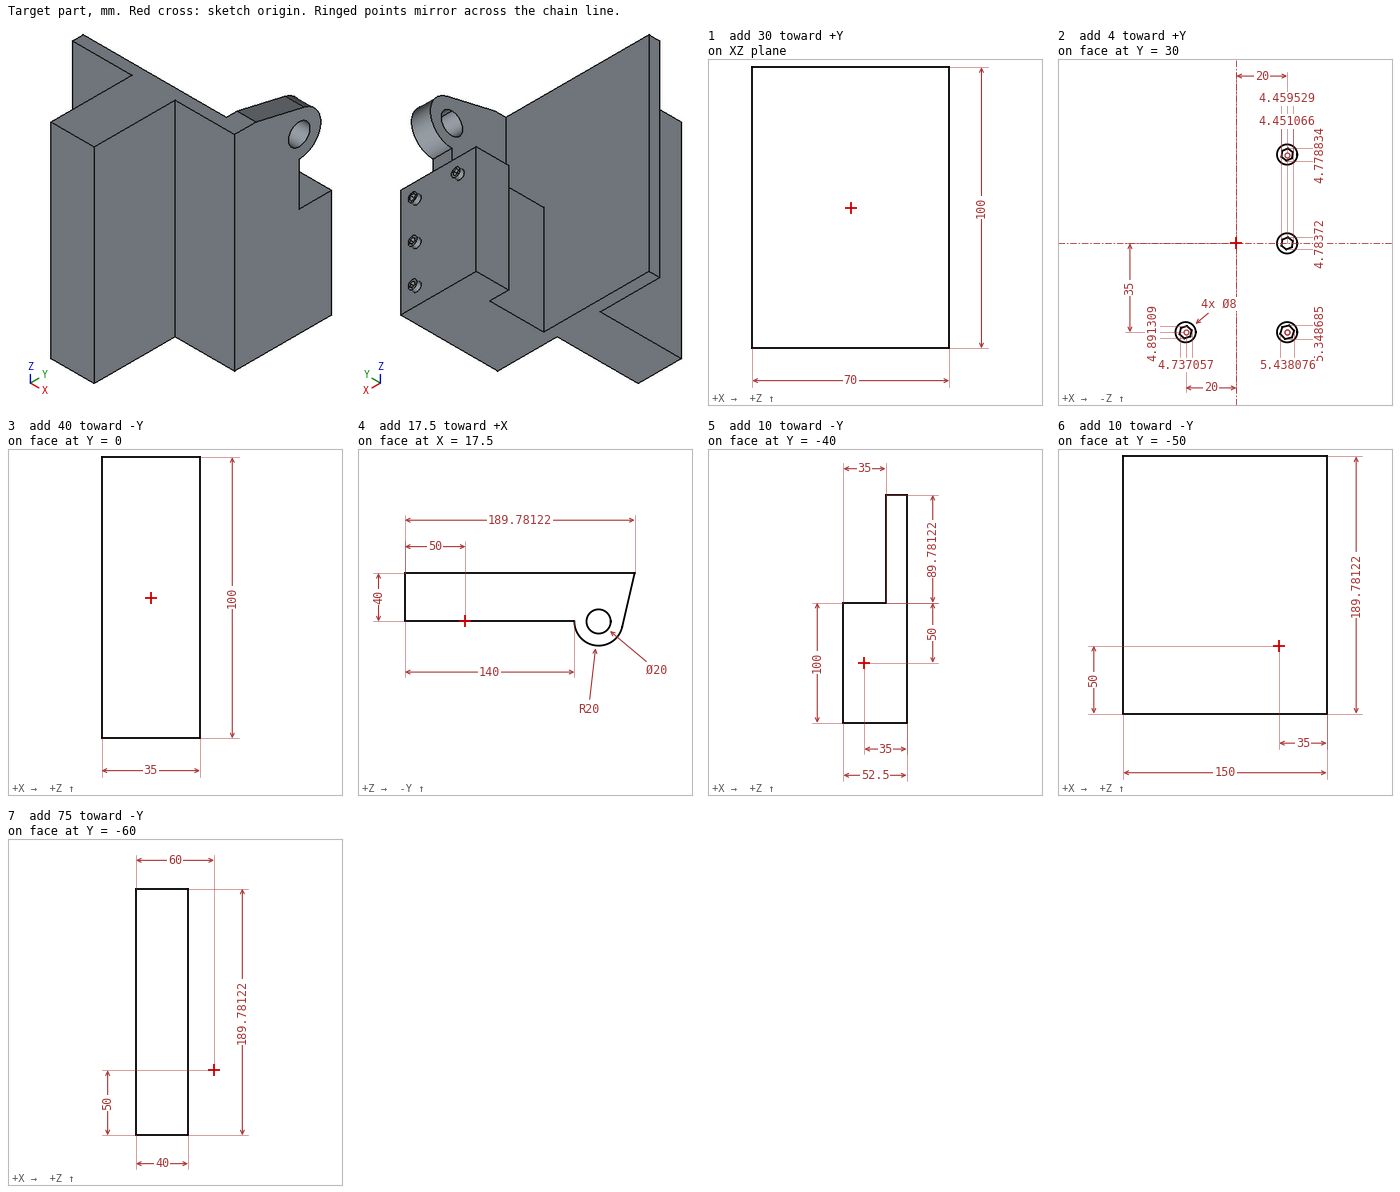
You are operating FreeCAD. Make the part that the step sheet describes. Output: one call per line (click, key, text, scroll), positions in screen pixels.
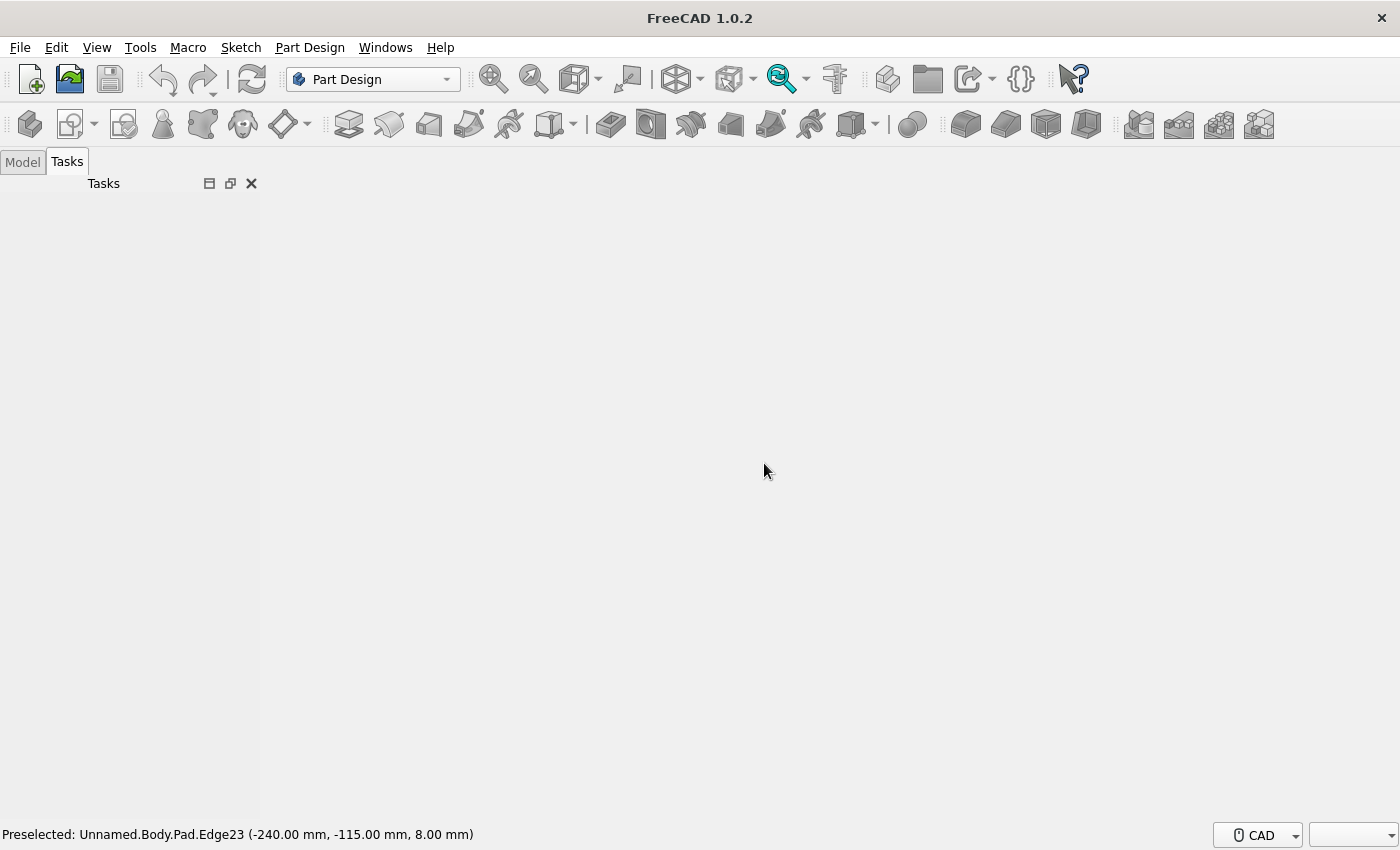
key(ctrl+n)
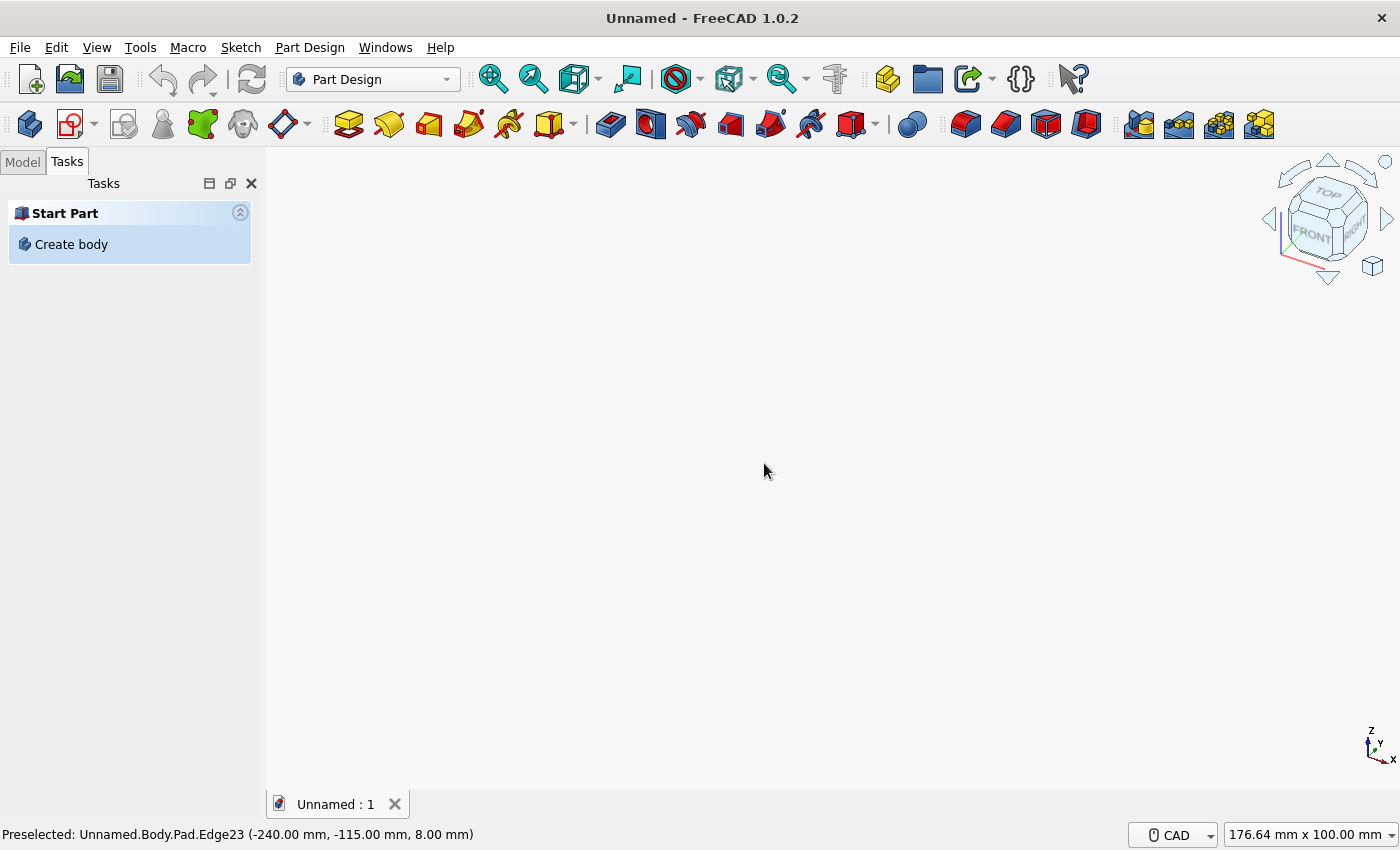
click(70, 124)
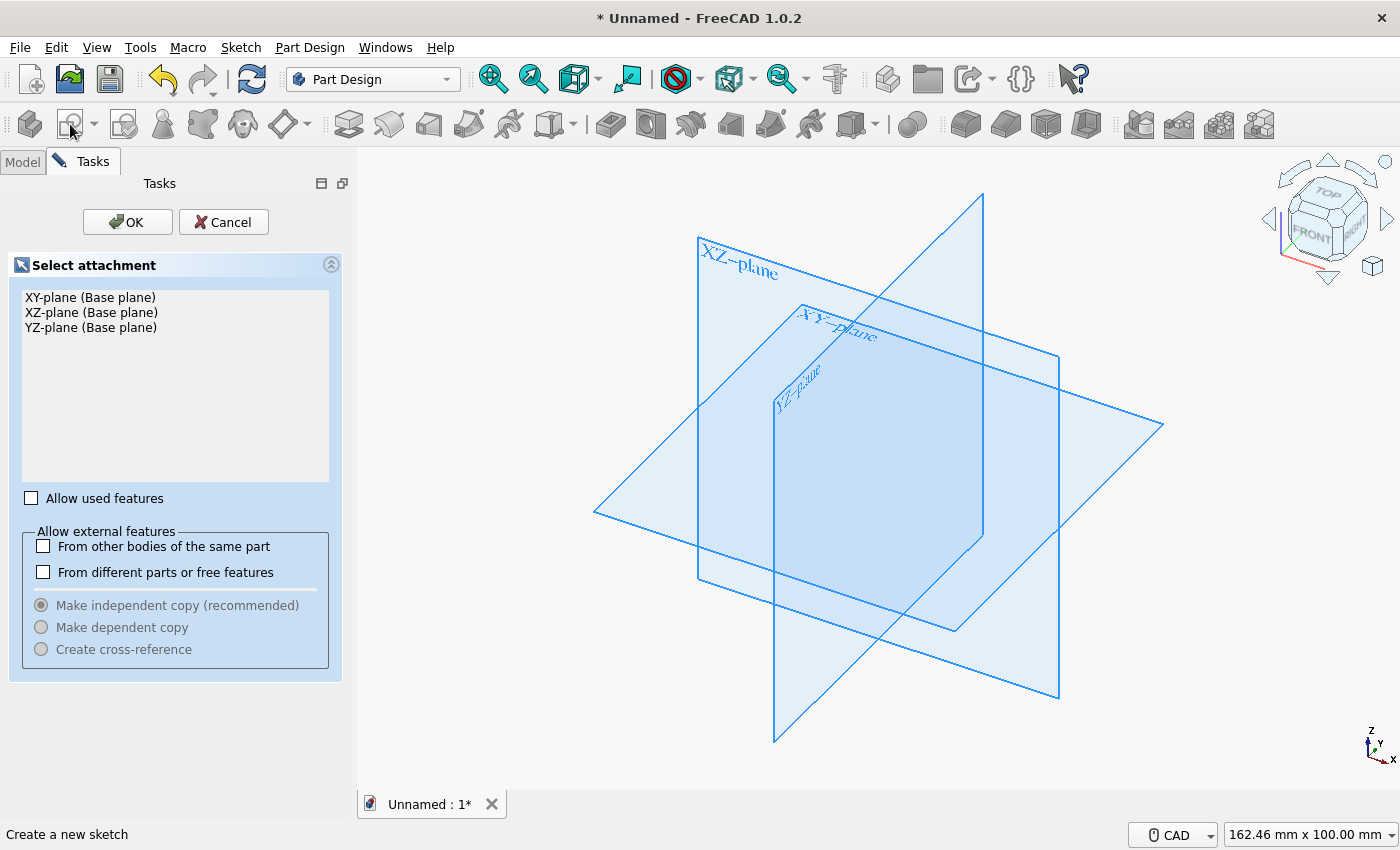
click(82, 312)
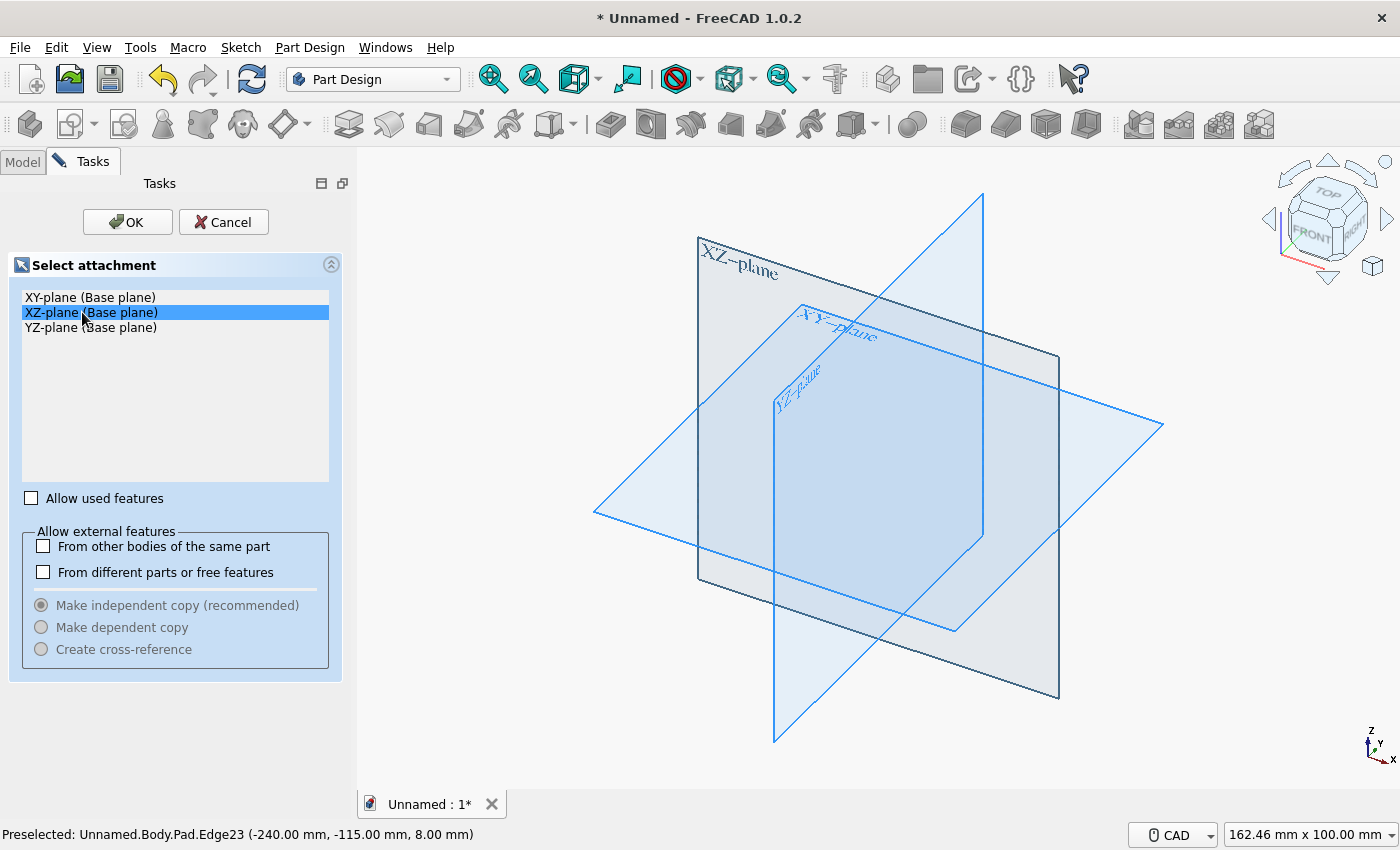
click(128, 222)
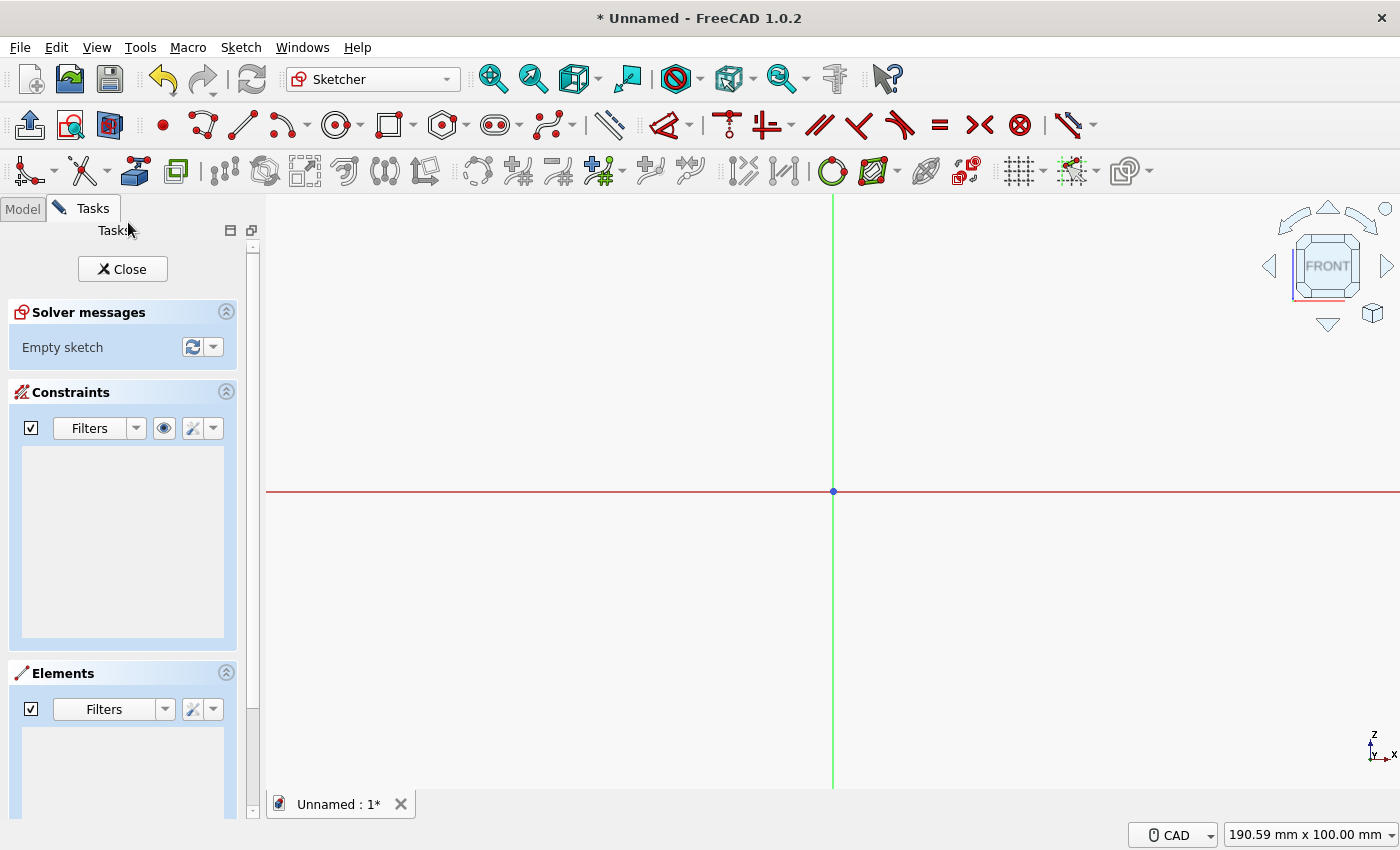
scroll(625, 492, down, 2)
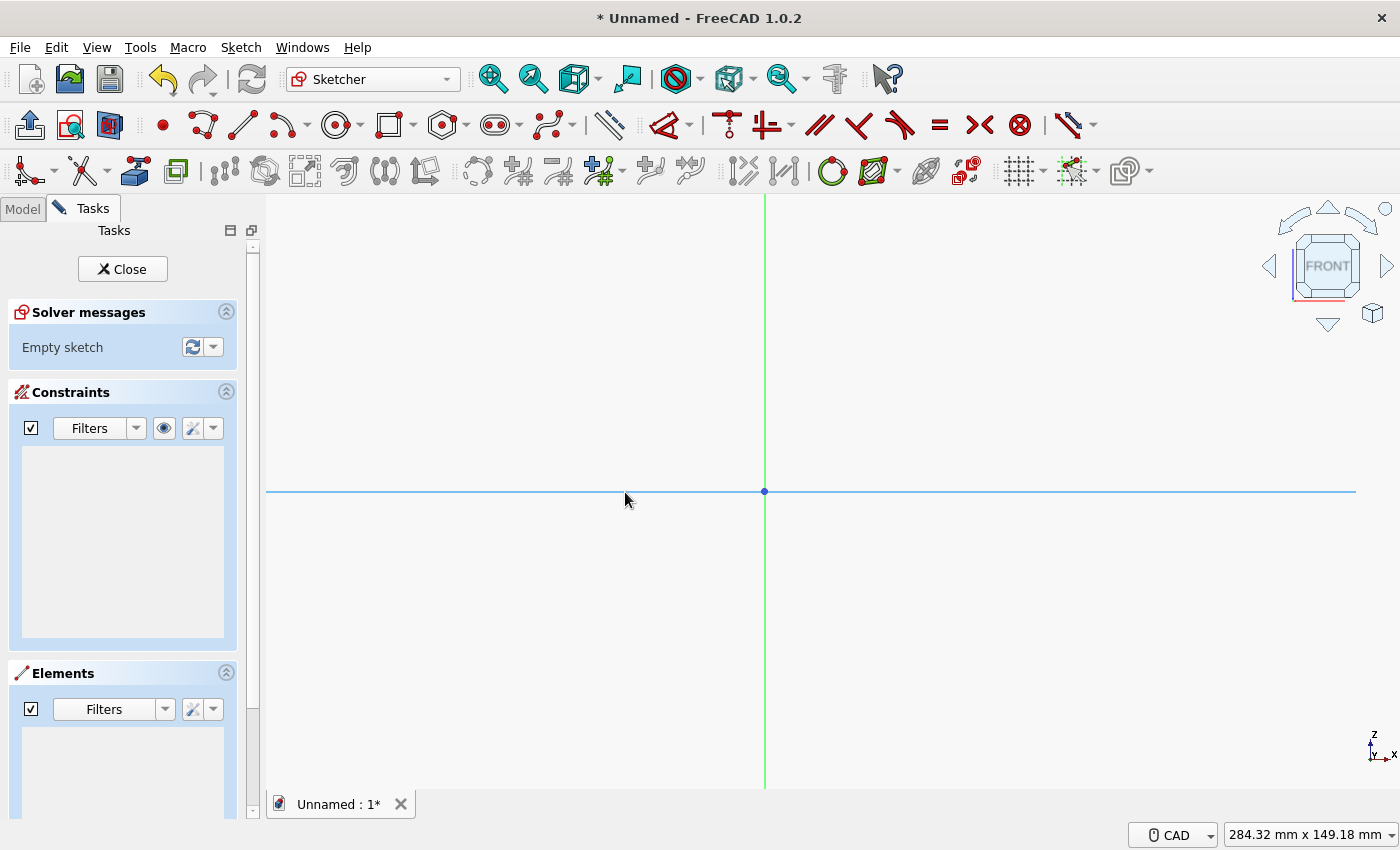
click(416, 126)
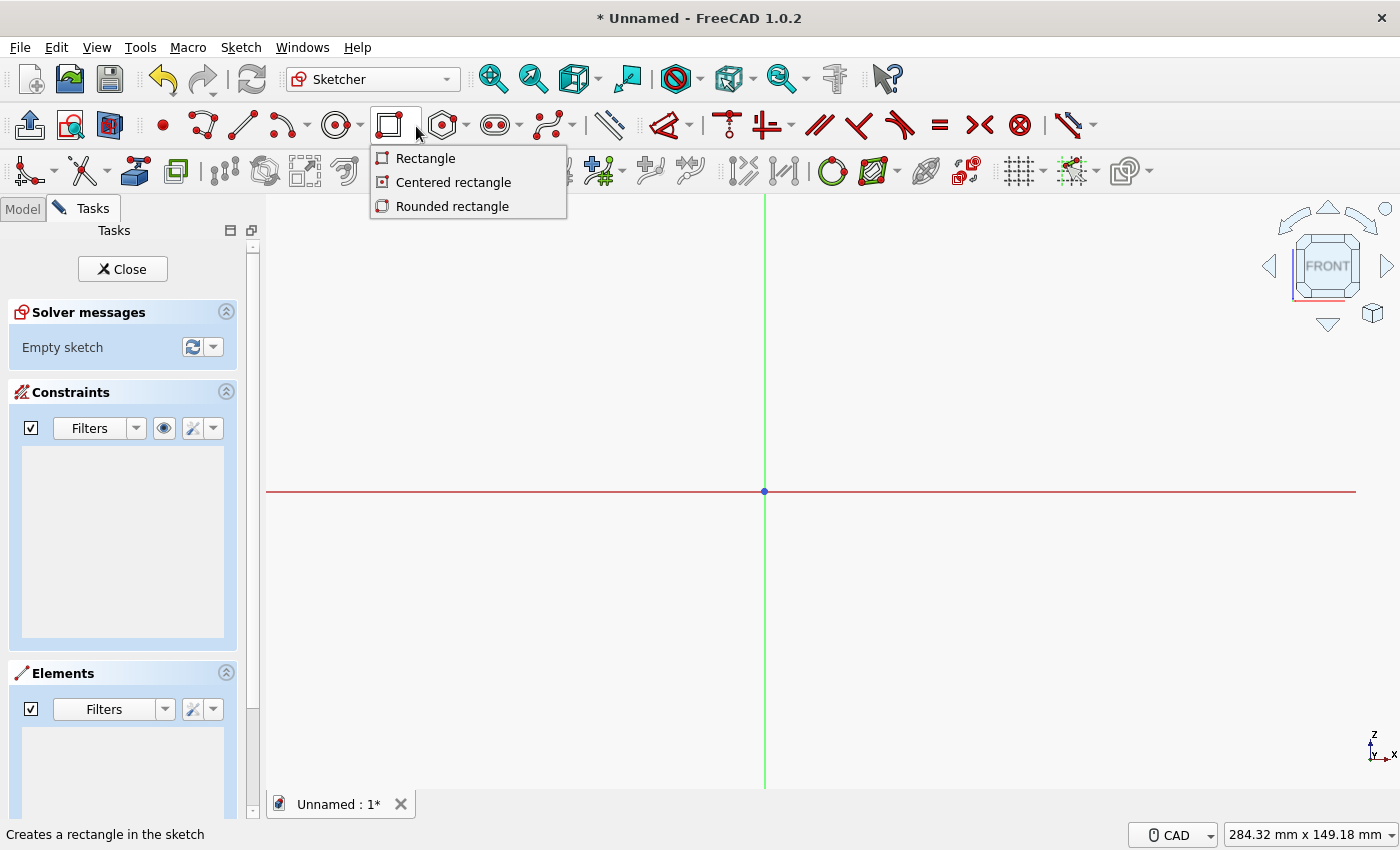
click(468, 182)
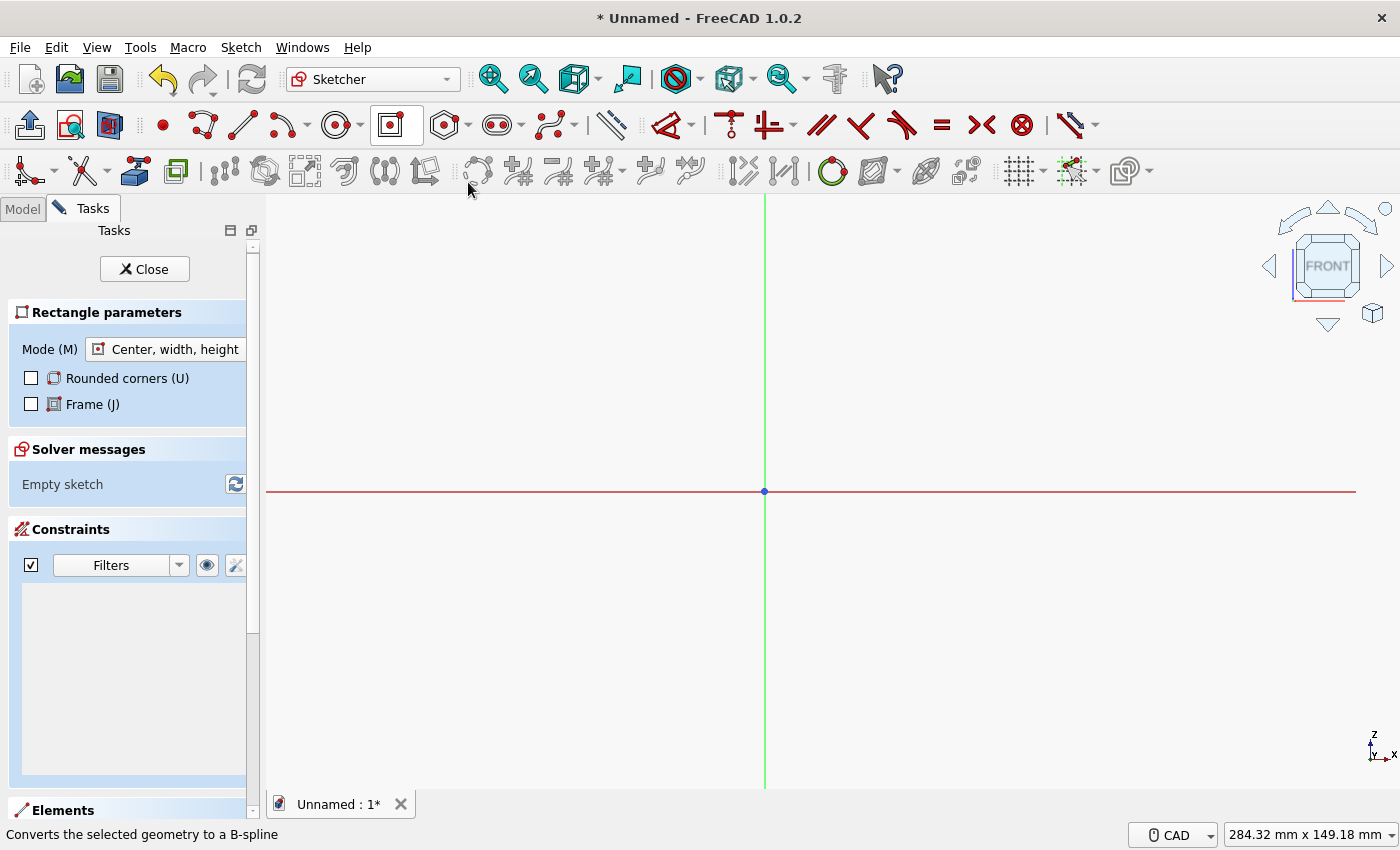
click(765, 492)
move(904, 292)